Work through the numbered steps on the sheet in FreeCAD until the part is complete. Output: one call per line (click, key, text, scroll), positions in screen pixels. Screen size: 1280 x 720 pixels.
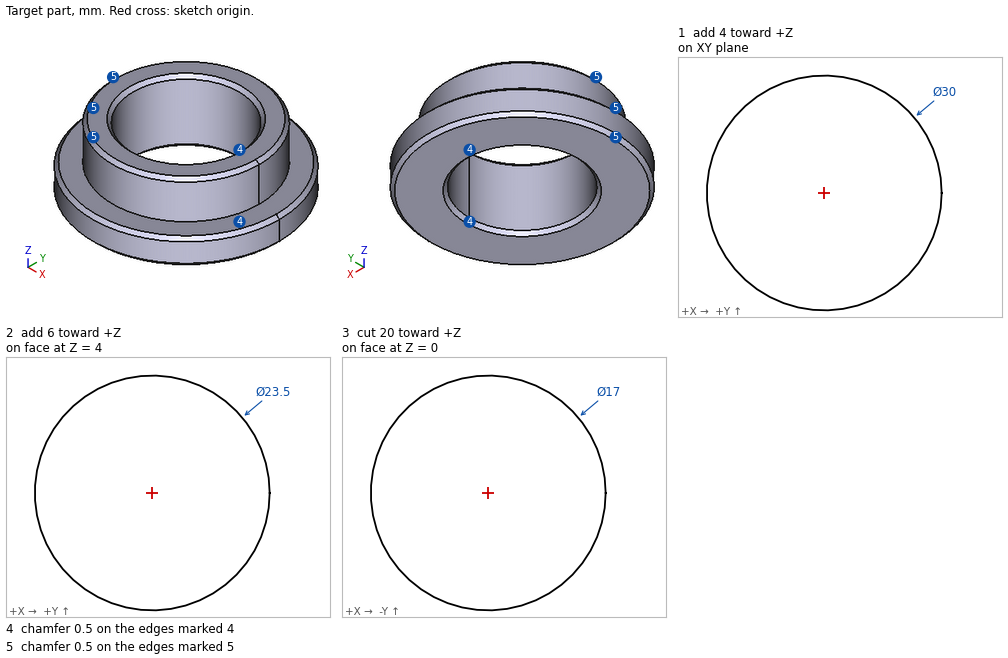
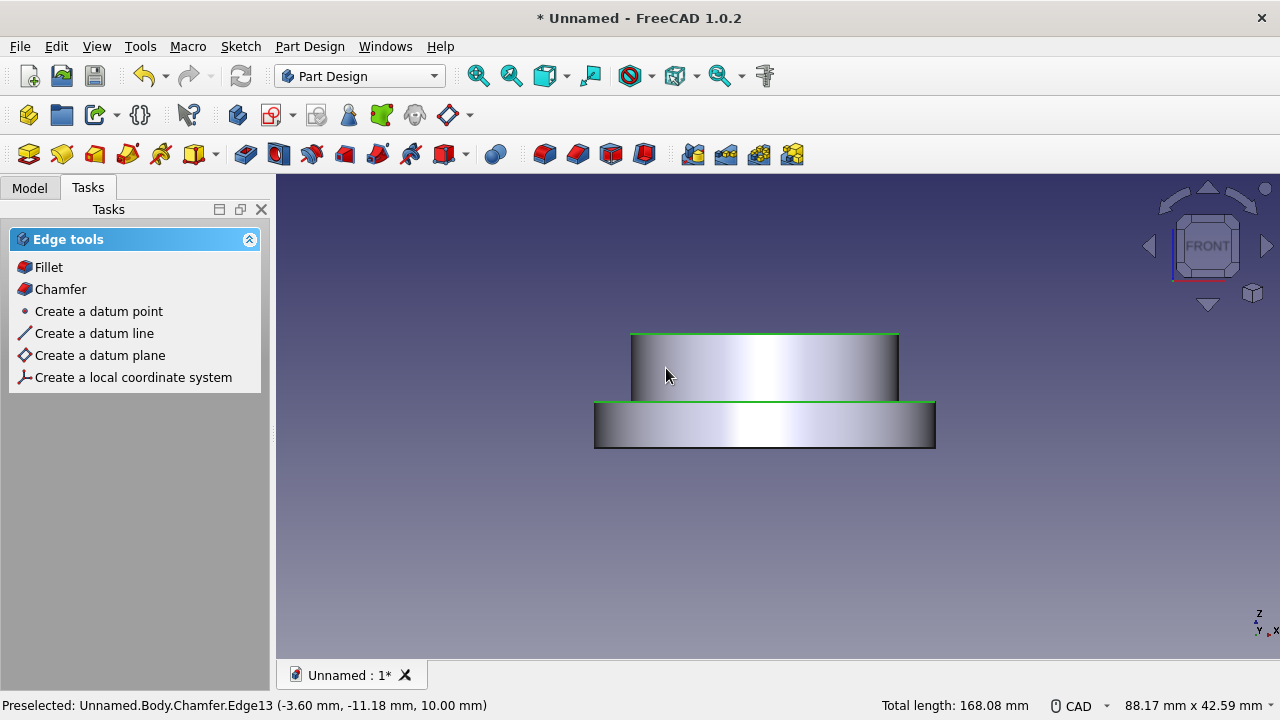
click(479, 76)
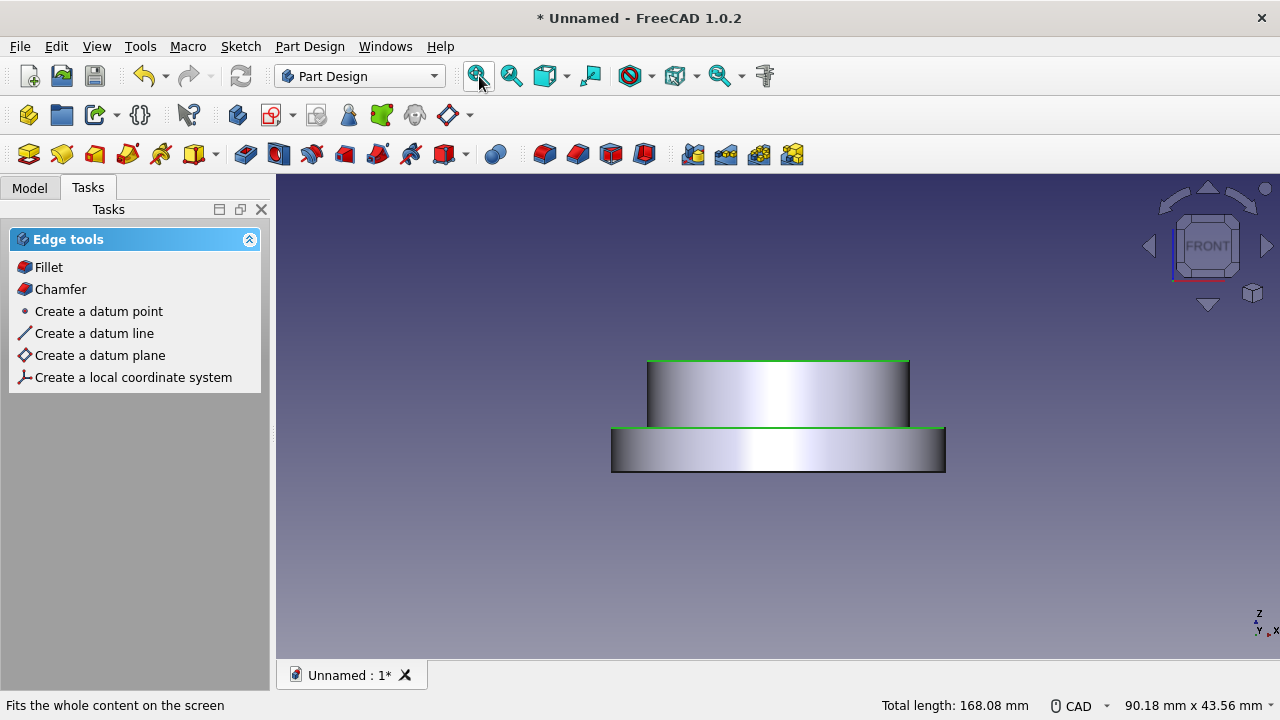
click(643, 471, ctrl)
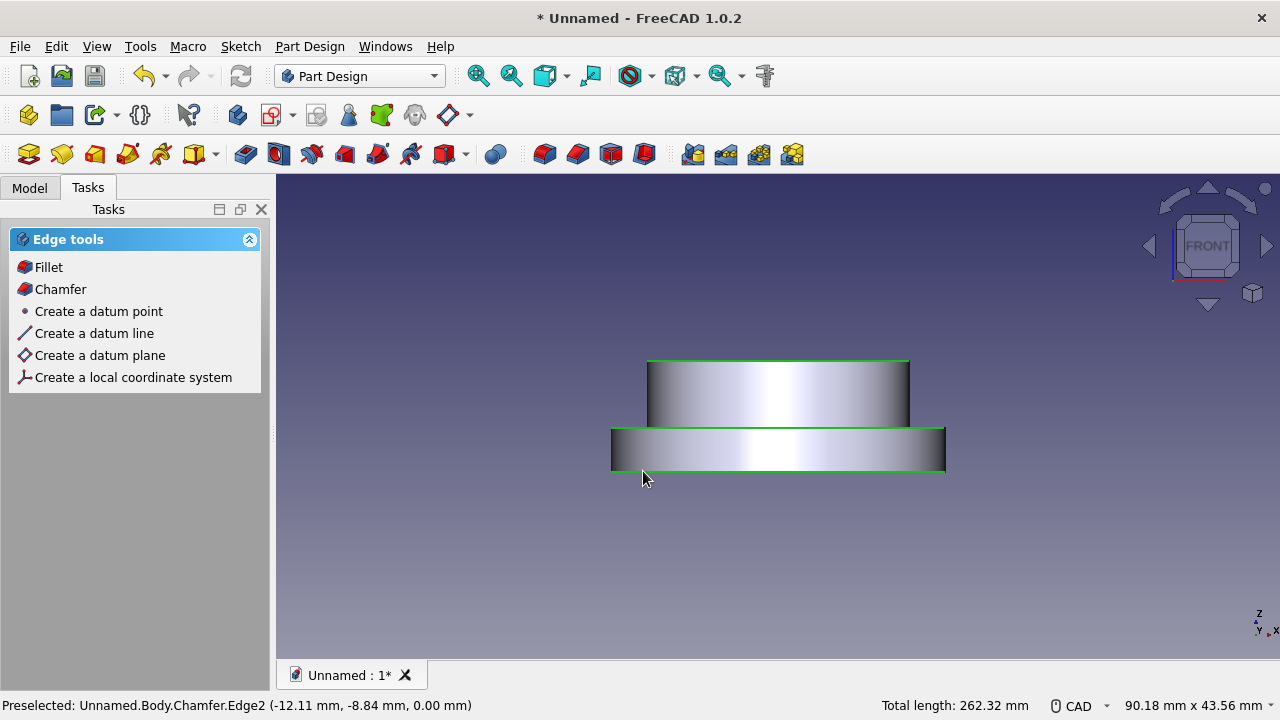
click(578, 154)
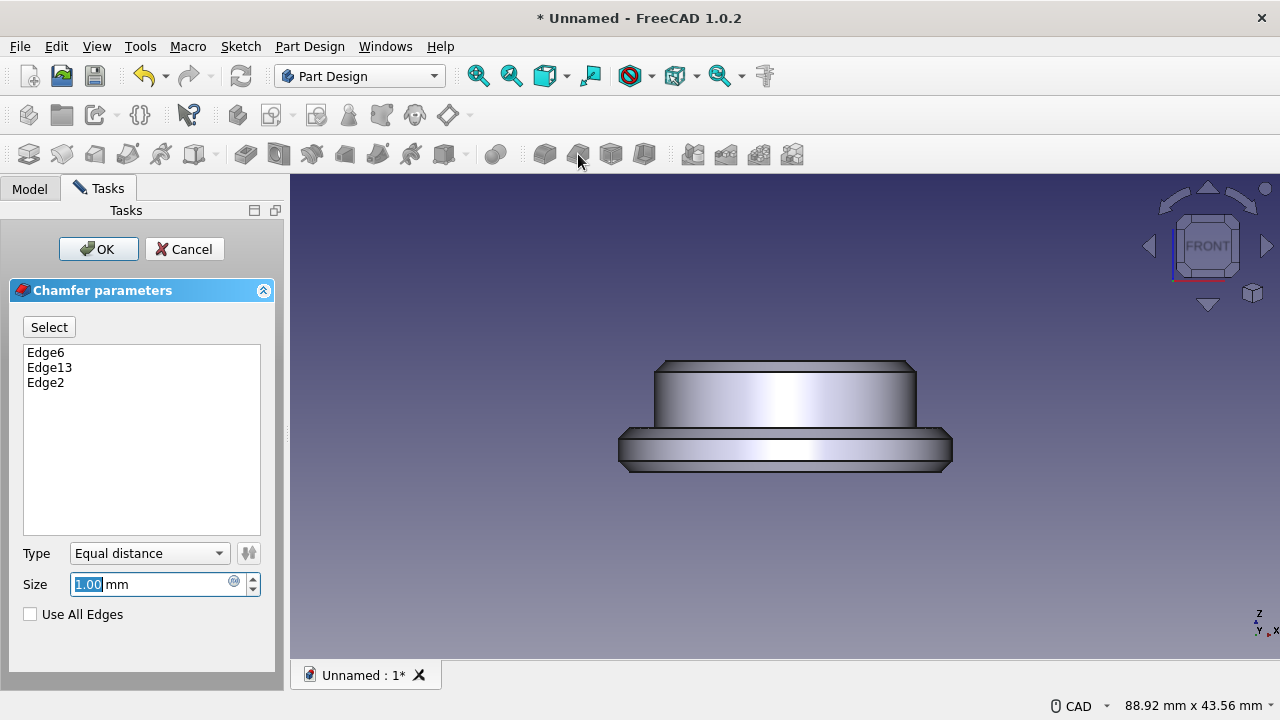
text(0.5)
key(Tab)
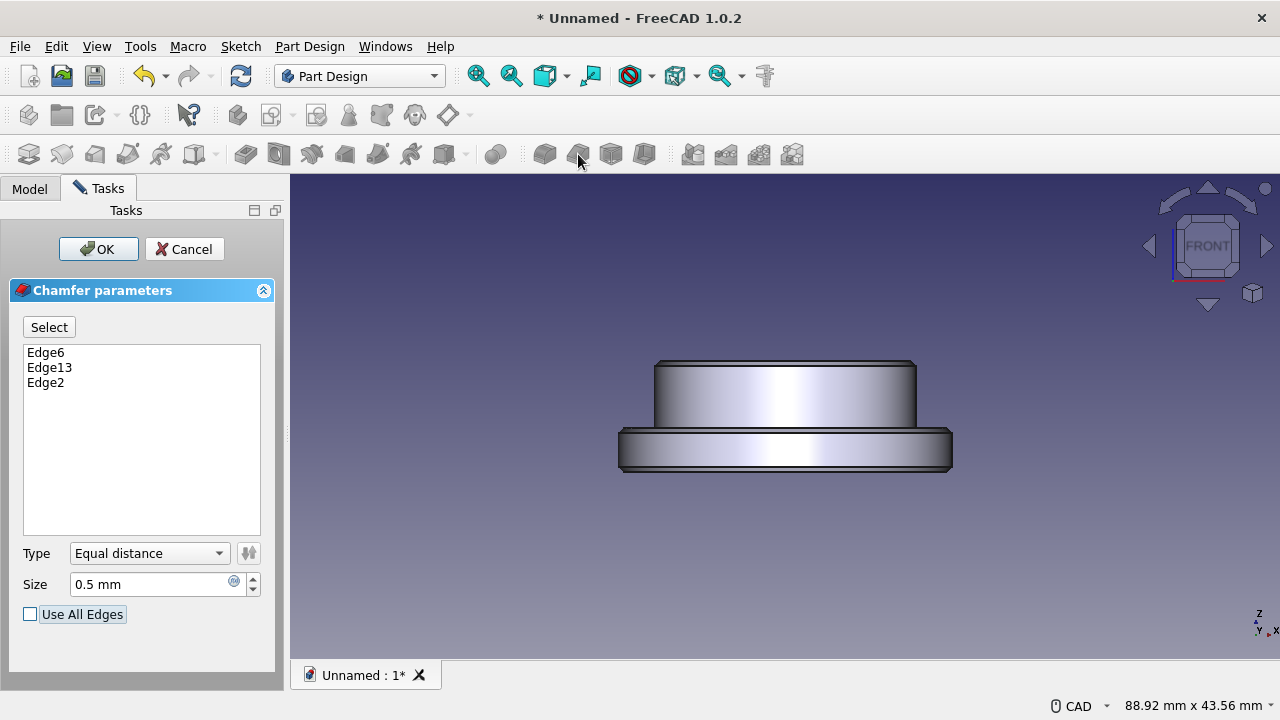
click(99, 249)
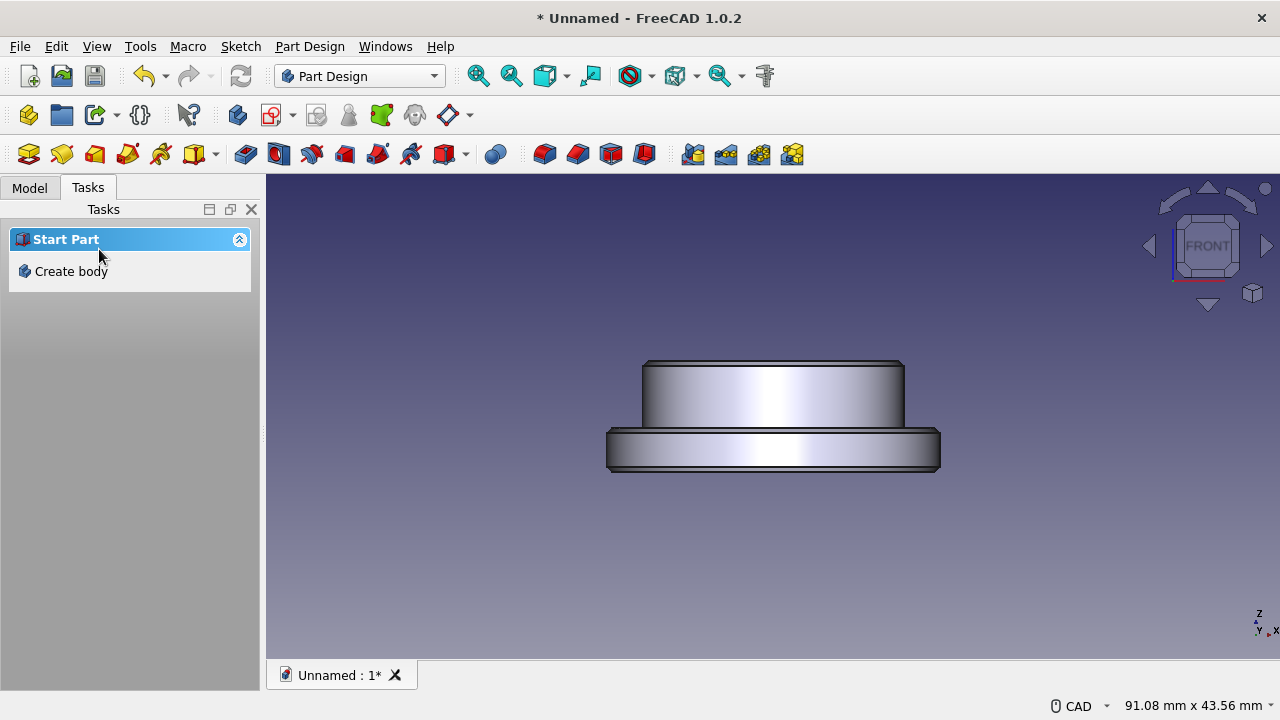
key(0)